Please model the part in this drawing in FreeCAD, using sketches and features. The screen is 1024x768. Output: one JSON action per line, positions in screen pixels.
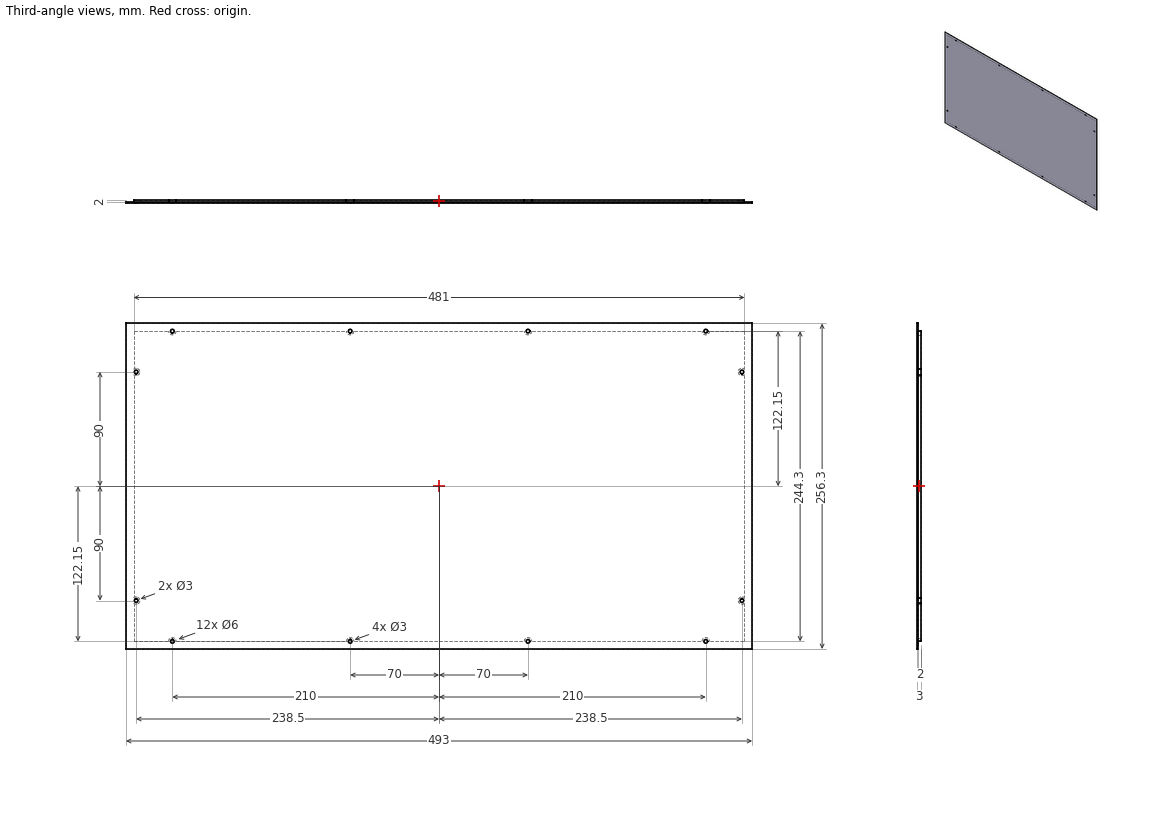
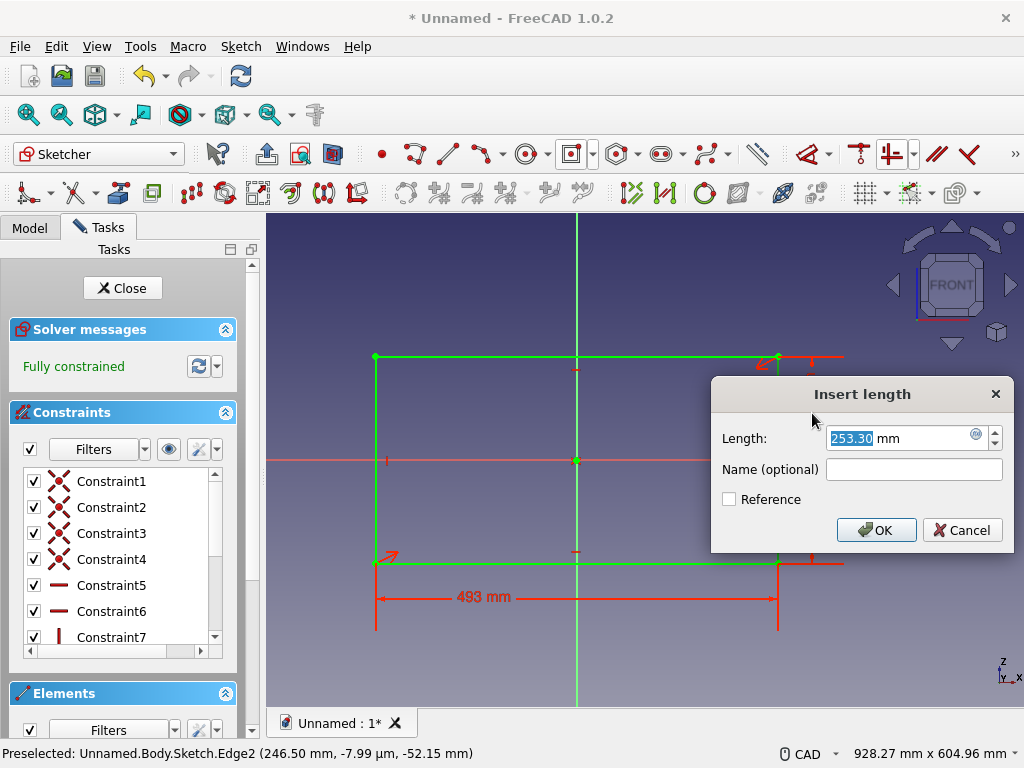
{"action": "type", "text": "256.3"}
{"action": "key", "text": "Return"}
{"action": "key", "text": "Escape"}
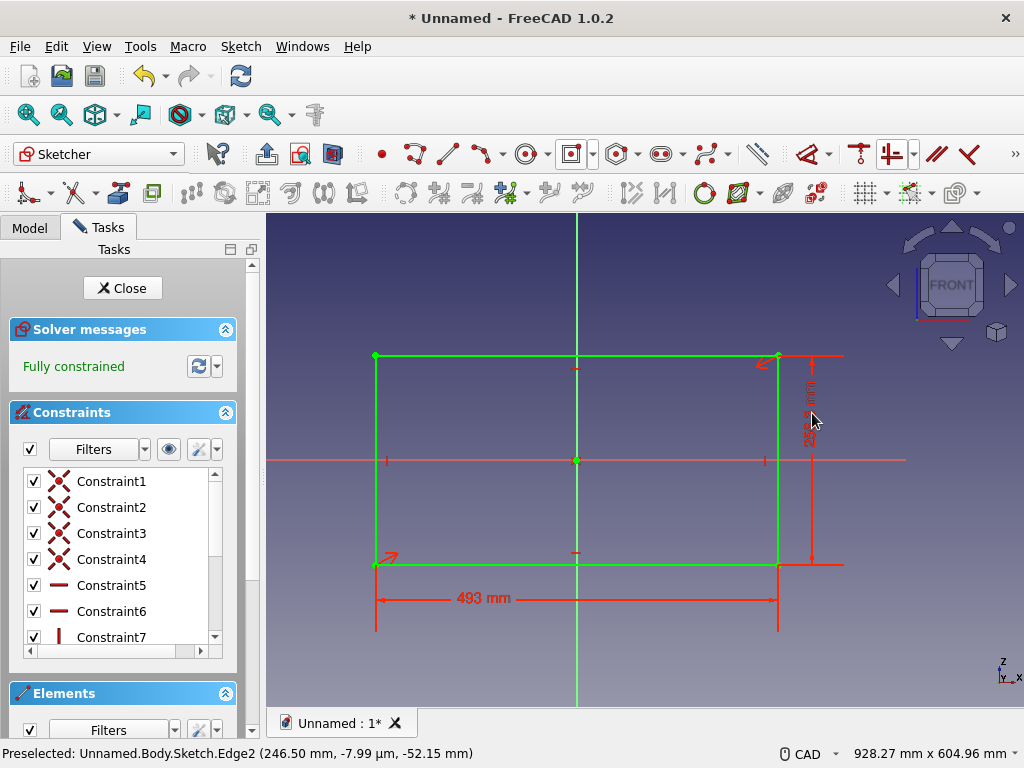
{"action": "left_click", "coordinate": [123, 288]}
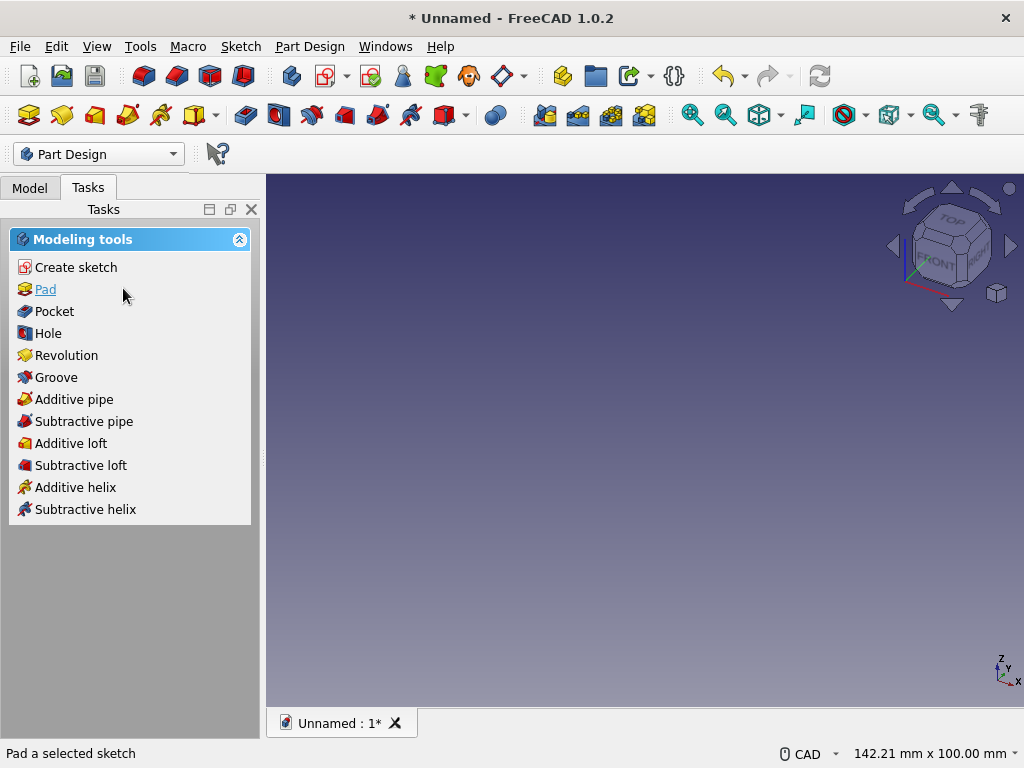
{"action": "left_click", "coordinate": [29, 116]}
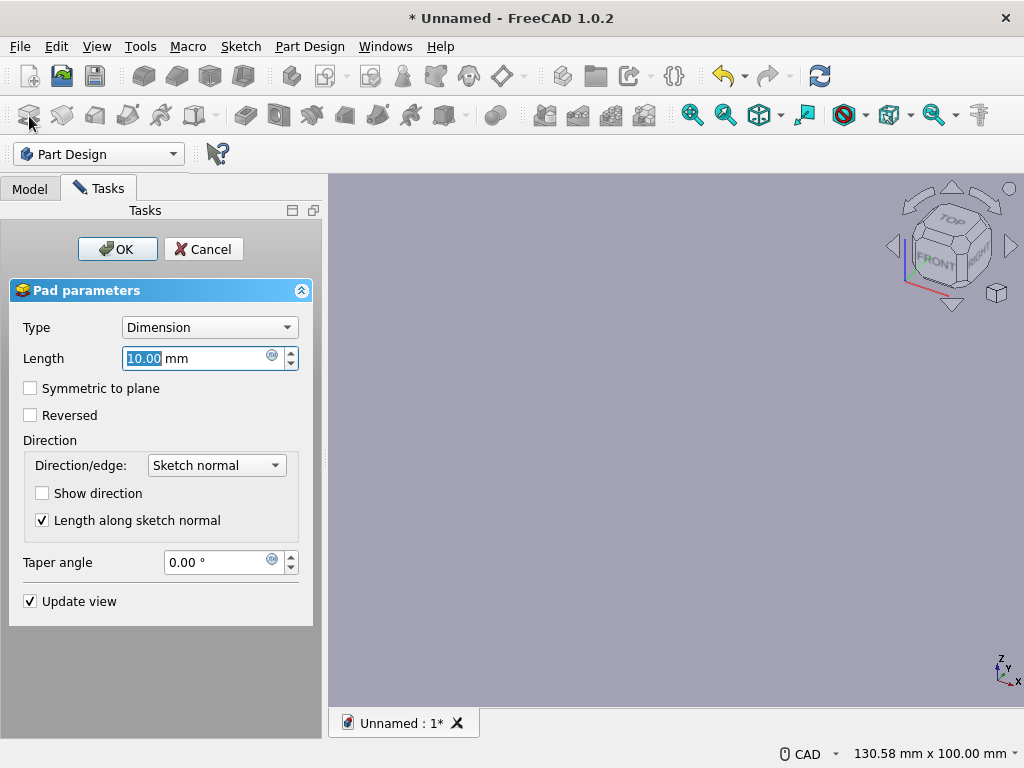
{"action": "type", "text": "3"}
{"action": "key", "text": "Tab"}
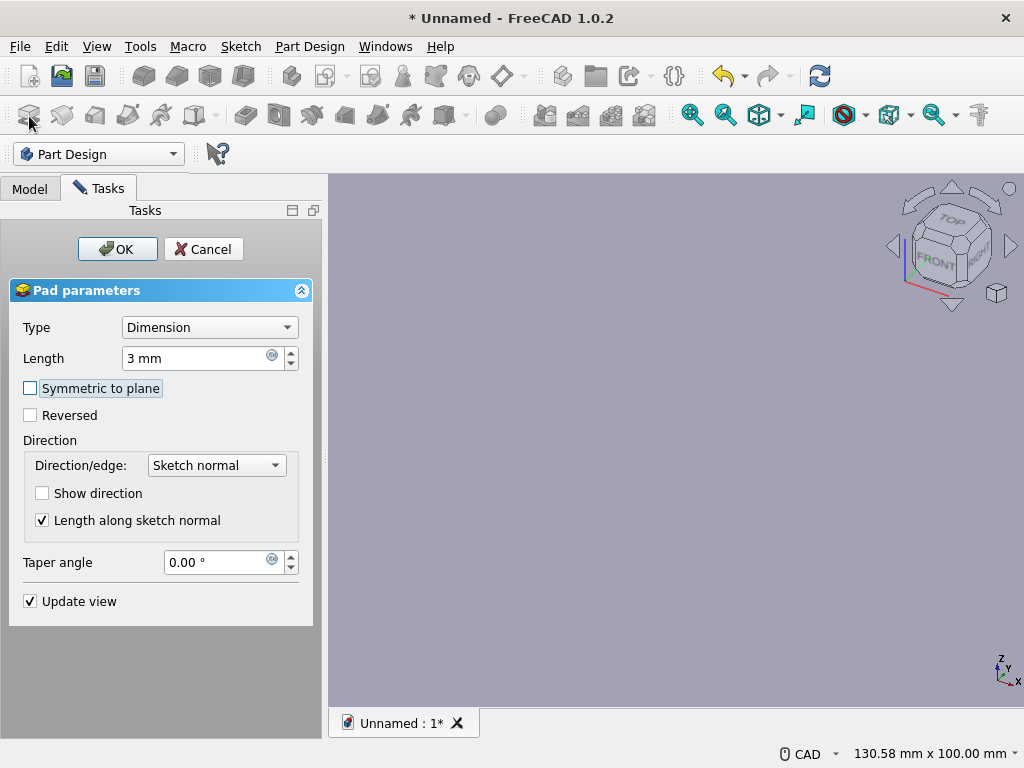
{"action": "left_click", "coordinate": [31, 388]}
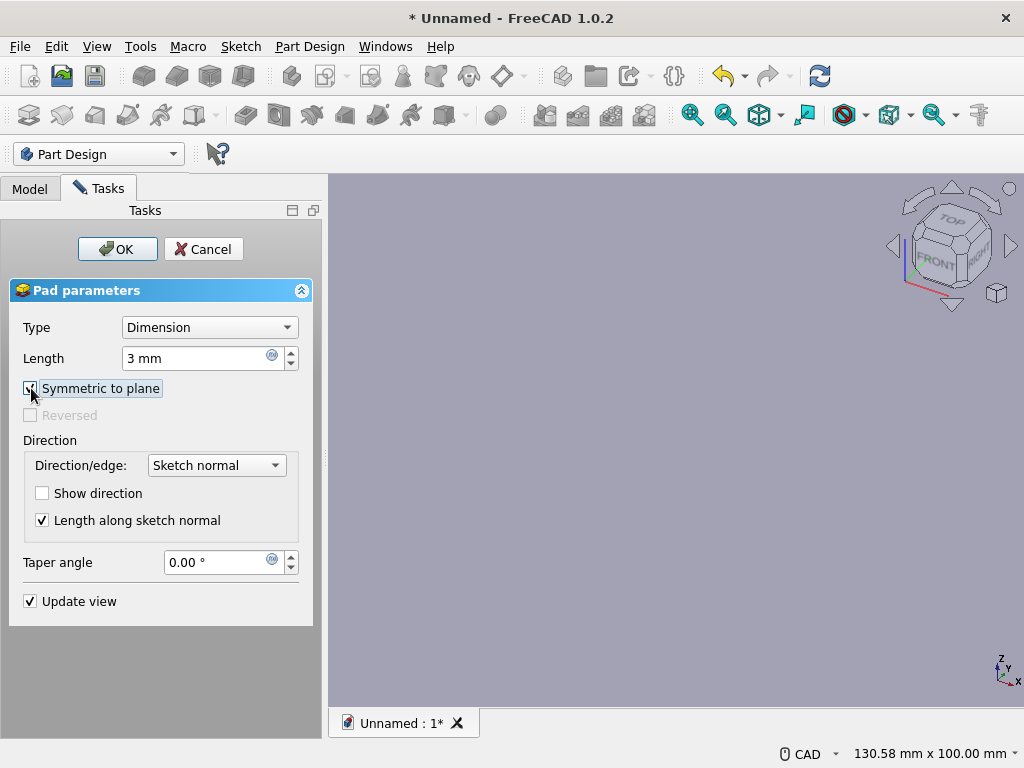
{"action": "left_click", "coordinate": [118, 249]}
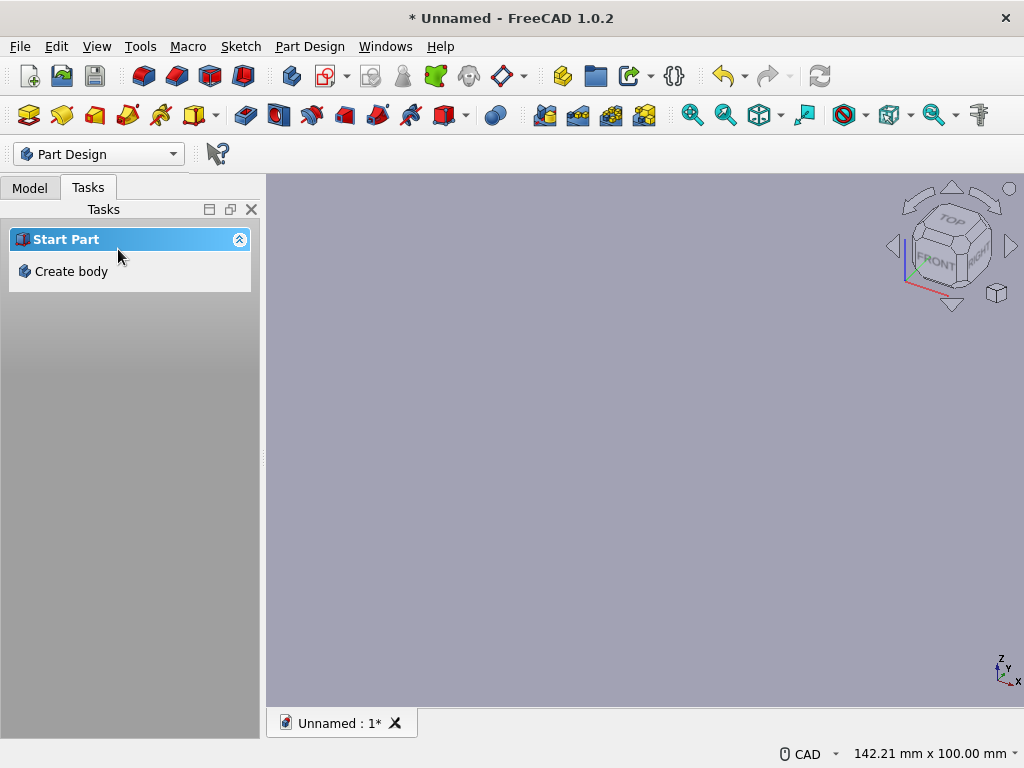
{"action": "left_click", "coordinate": [693, 116]}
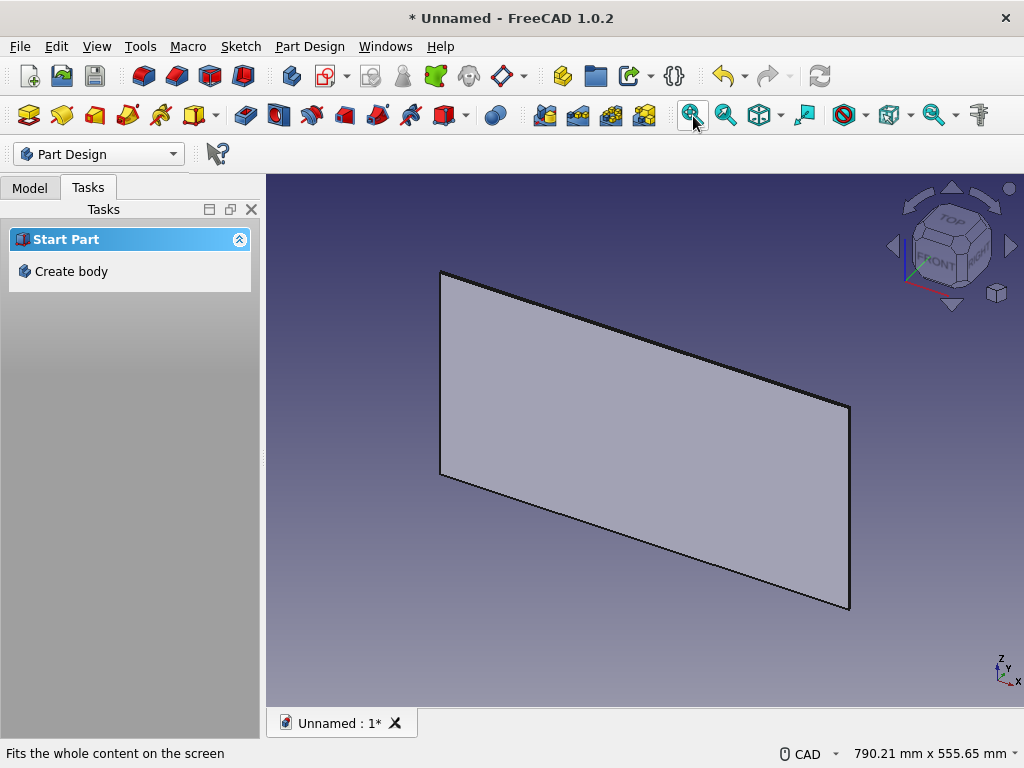
{"action": "key", "text": "4"}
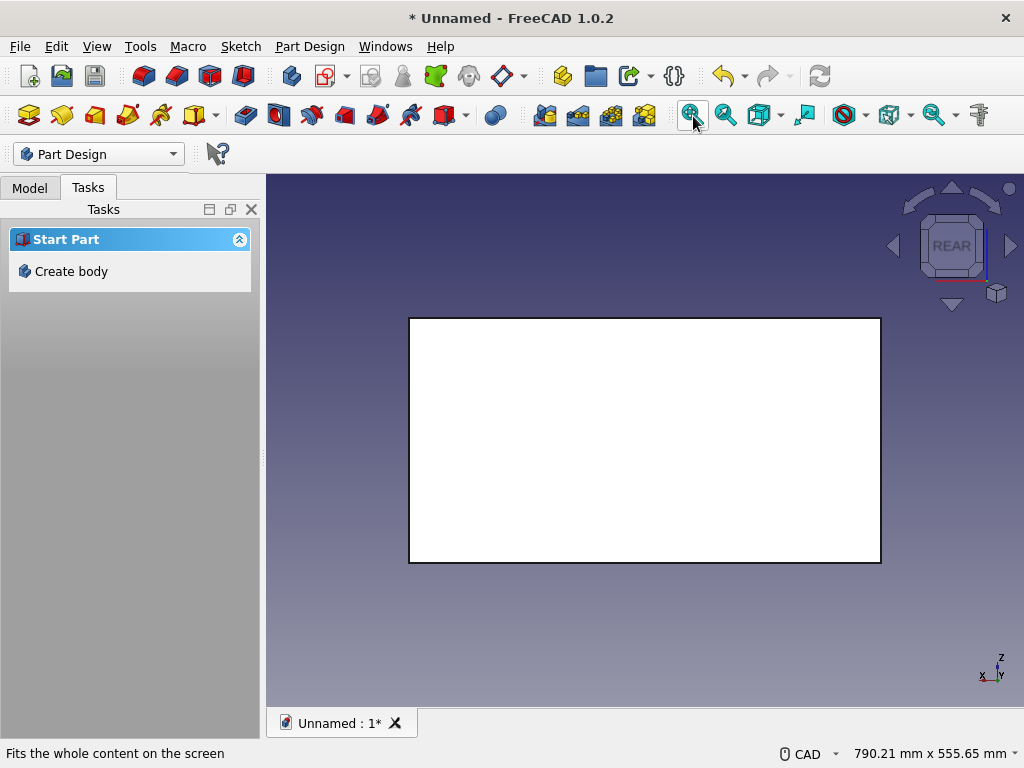
{"action": "left_click", "coordinate": [577, 440]}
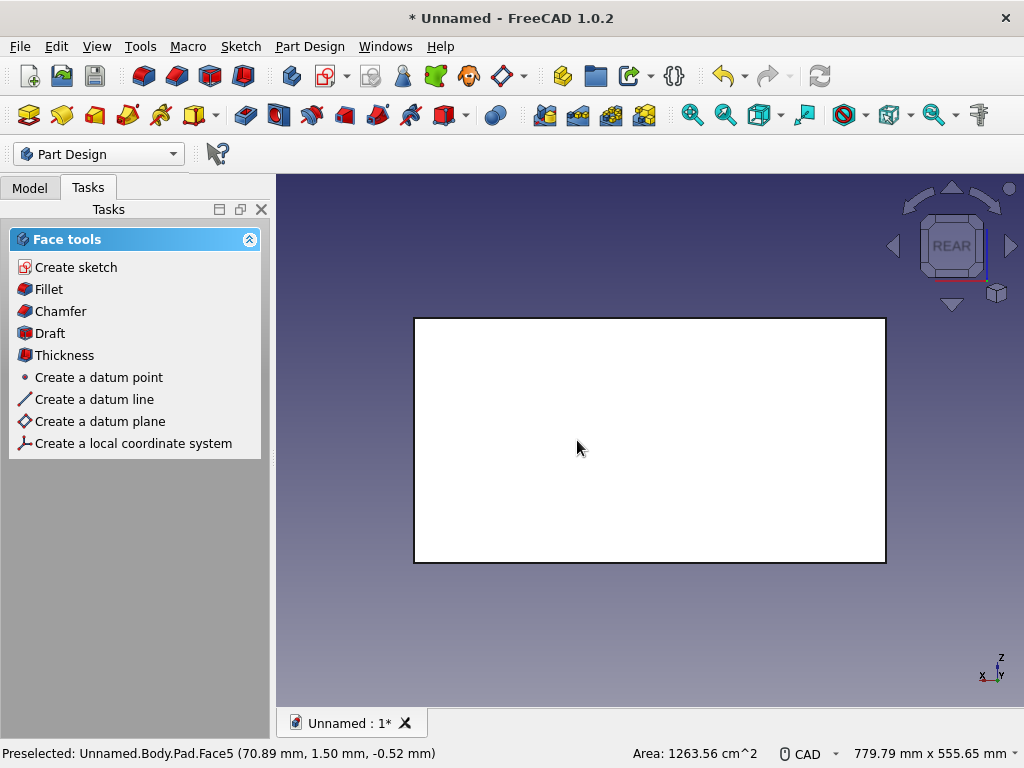
{"action": "left_click", "coordinate": [324, 76]}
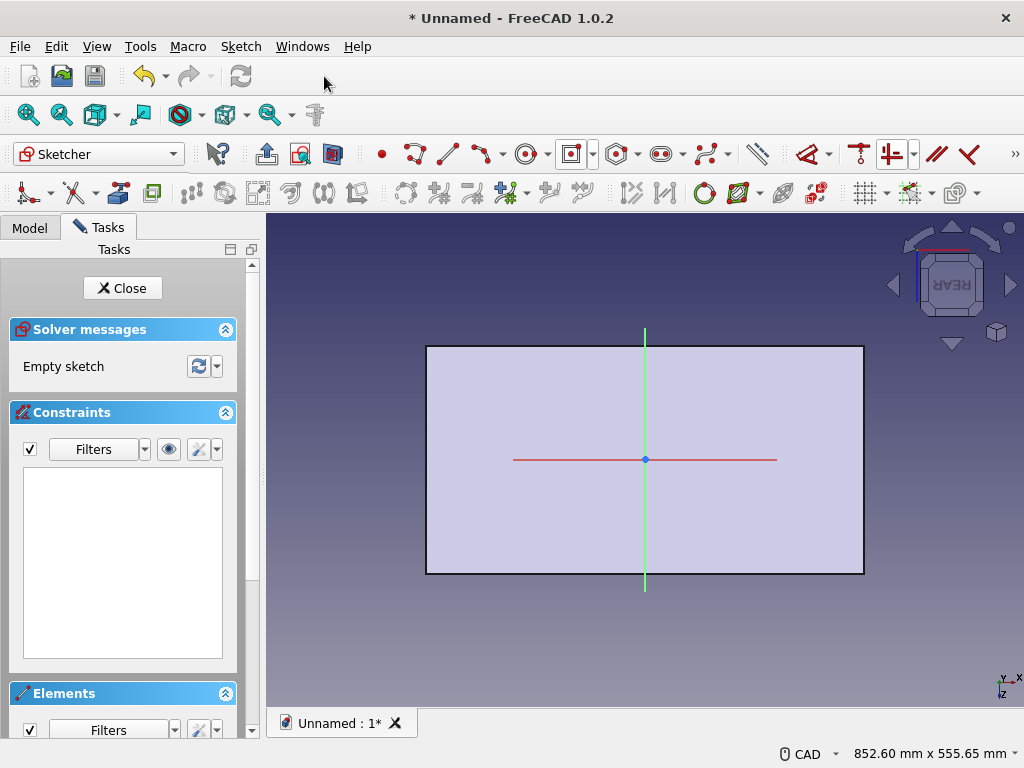
{"action": "scroll", "coordinate": [294, 460], "scroll_direction": "down", "scroll_amount": 1}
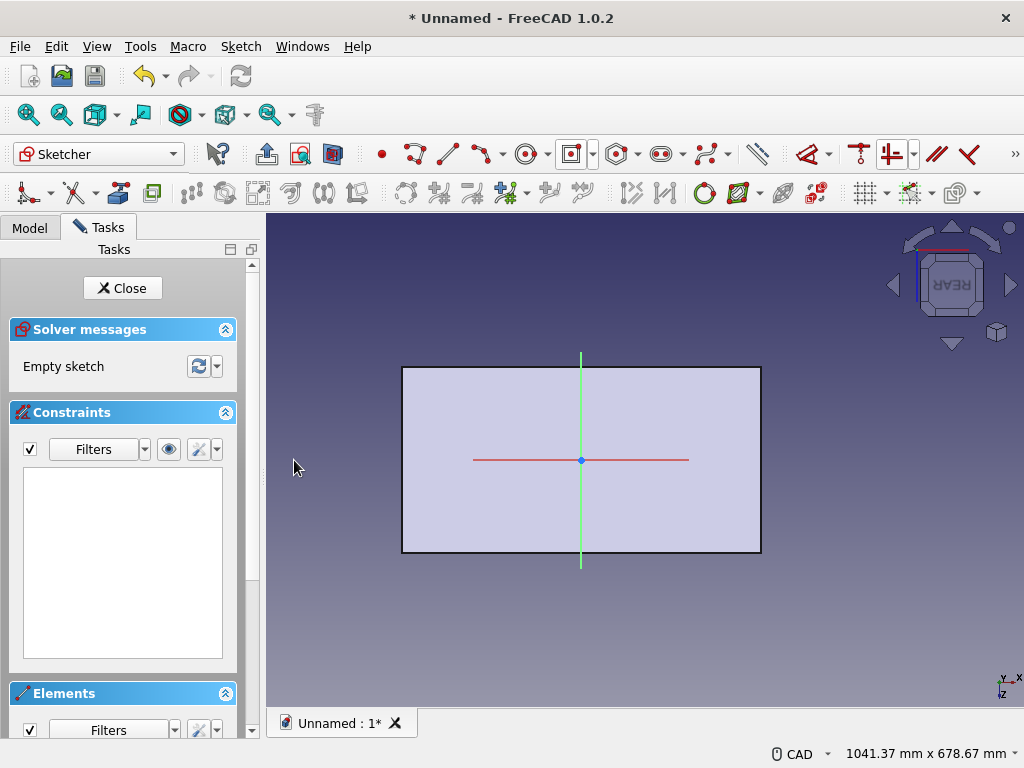
{"action": "left_click", "coordinate": [570, 154]}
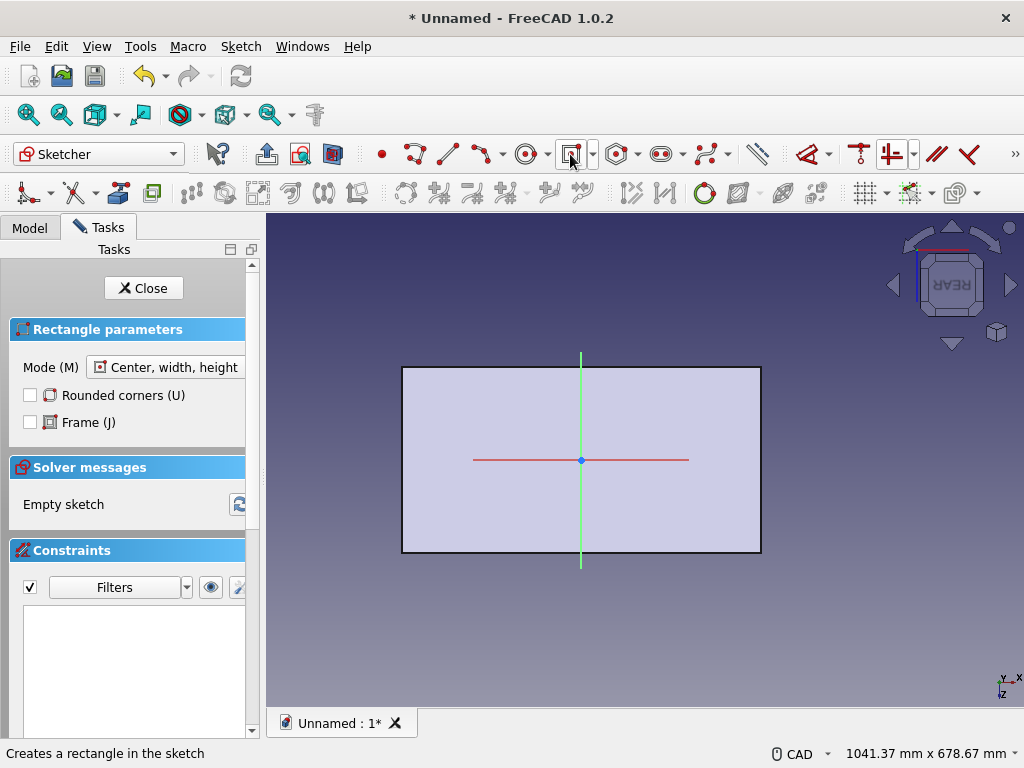
{"action": "left_click", "coordinate": [581, 460]}
{"action": "left_click", "coordinate": [761, 367]}